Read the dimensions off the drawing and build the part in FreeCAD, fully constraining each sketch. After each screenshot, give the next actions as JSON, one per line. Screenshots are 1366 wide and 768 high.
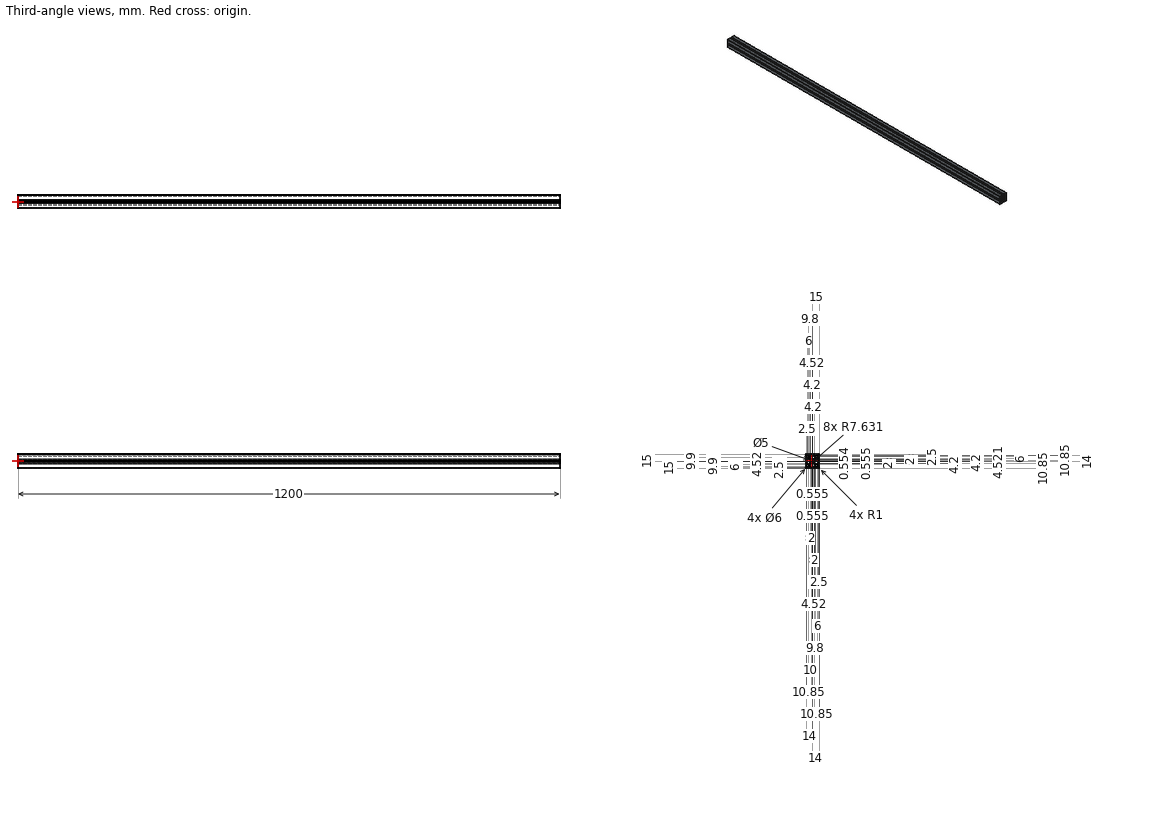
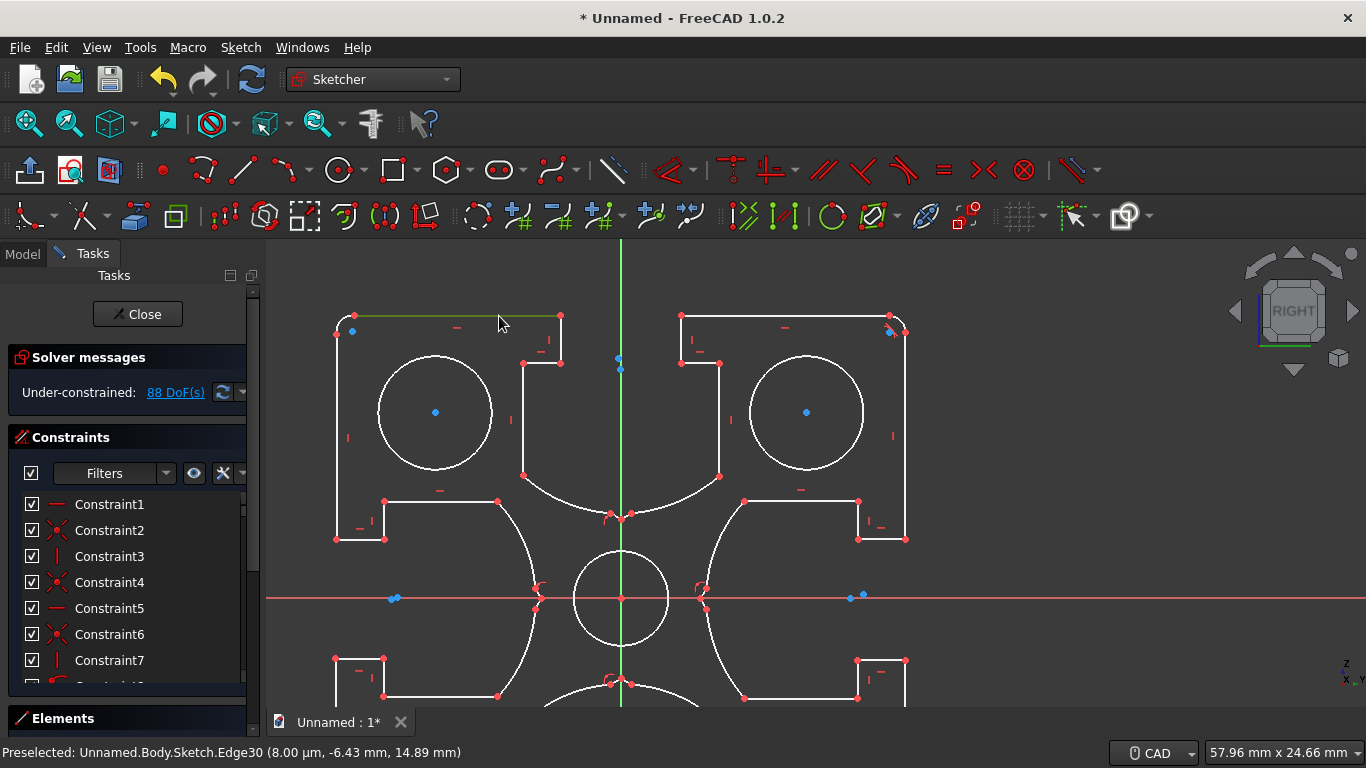
{"action": "left_click", "coordinate": [341, 320]}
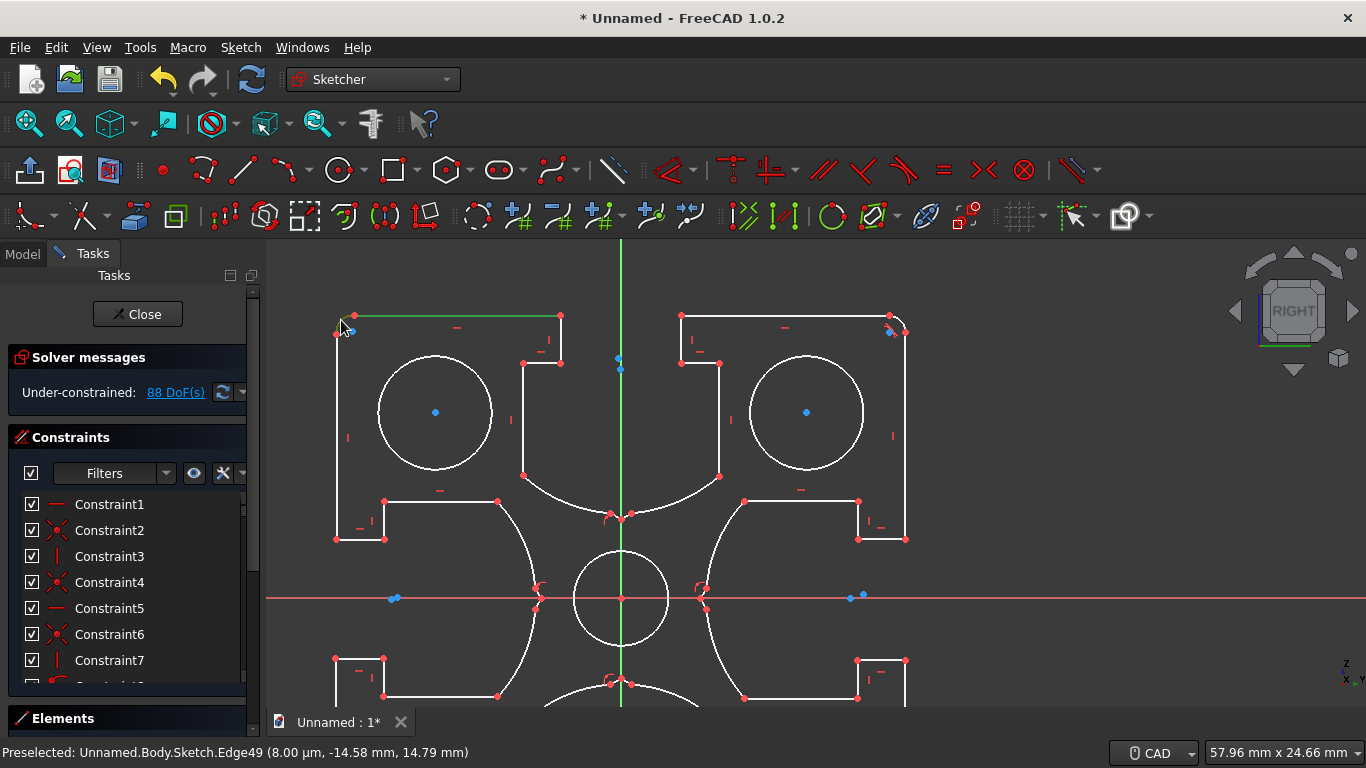
{"action": "left_click", "coordinate": [904, 170]}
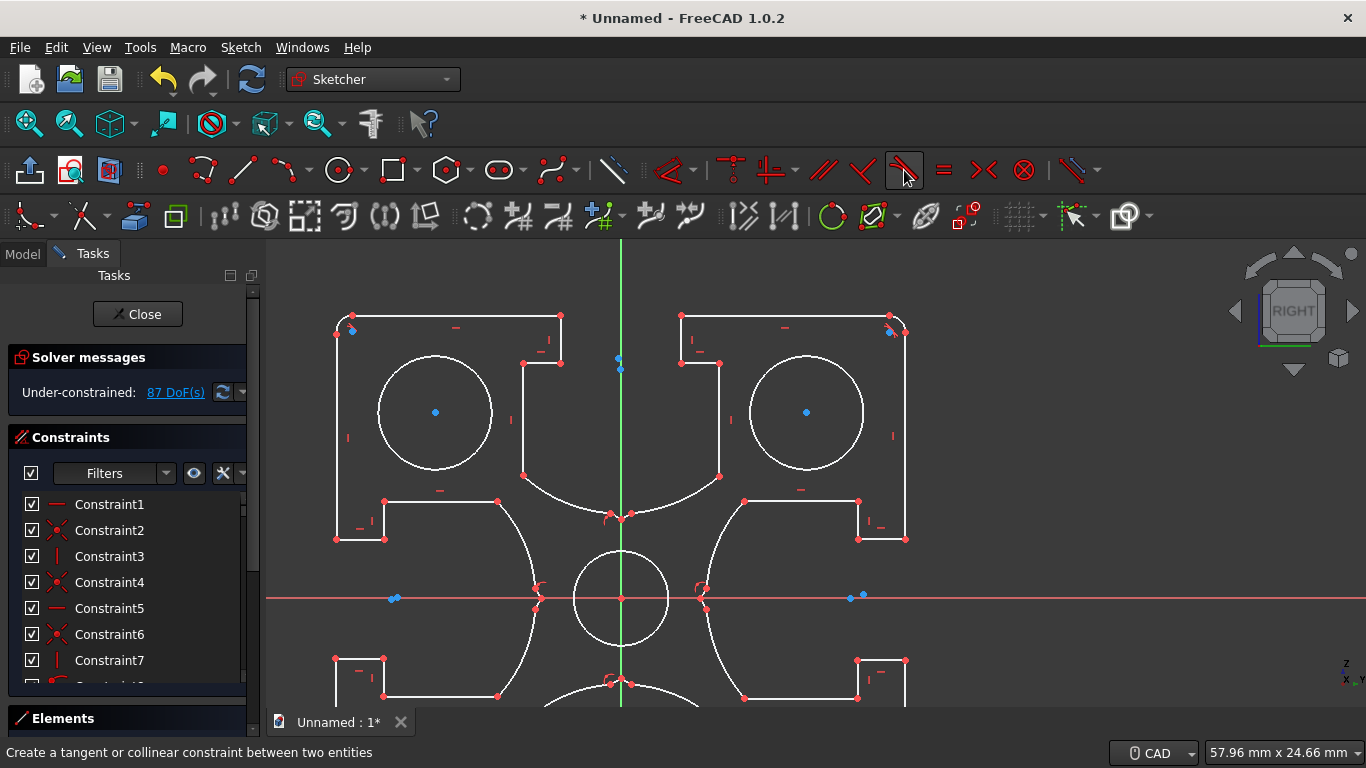
{"action": "left_click", "coordinate": [337, 396]}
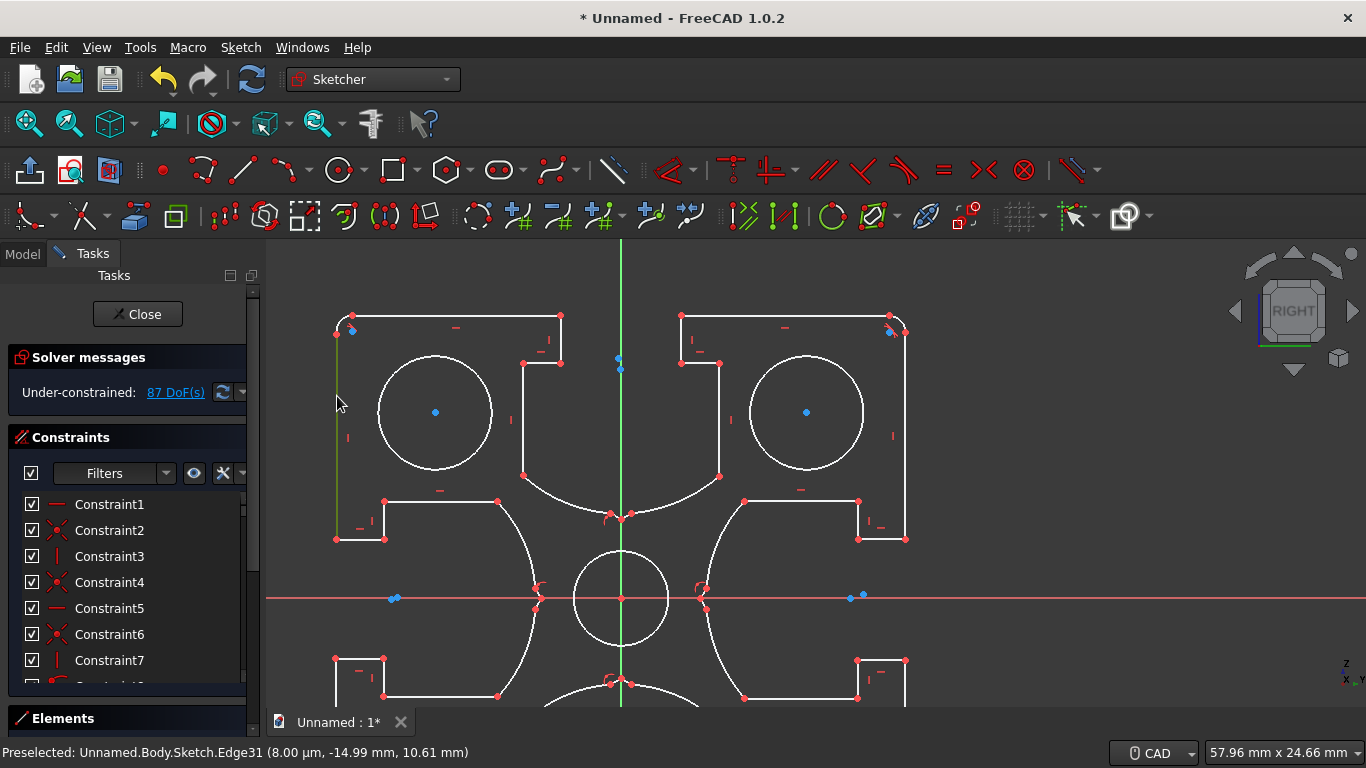
{"action": "left_click", "coordinate": [340, 321]}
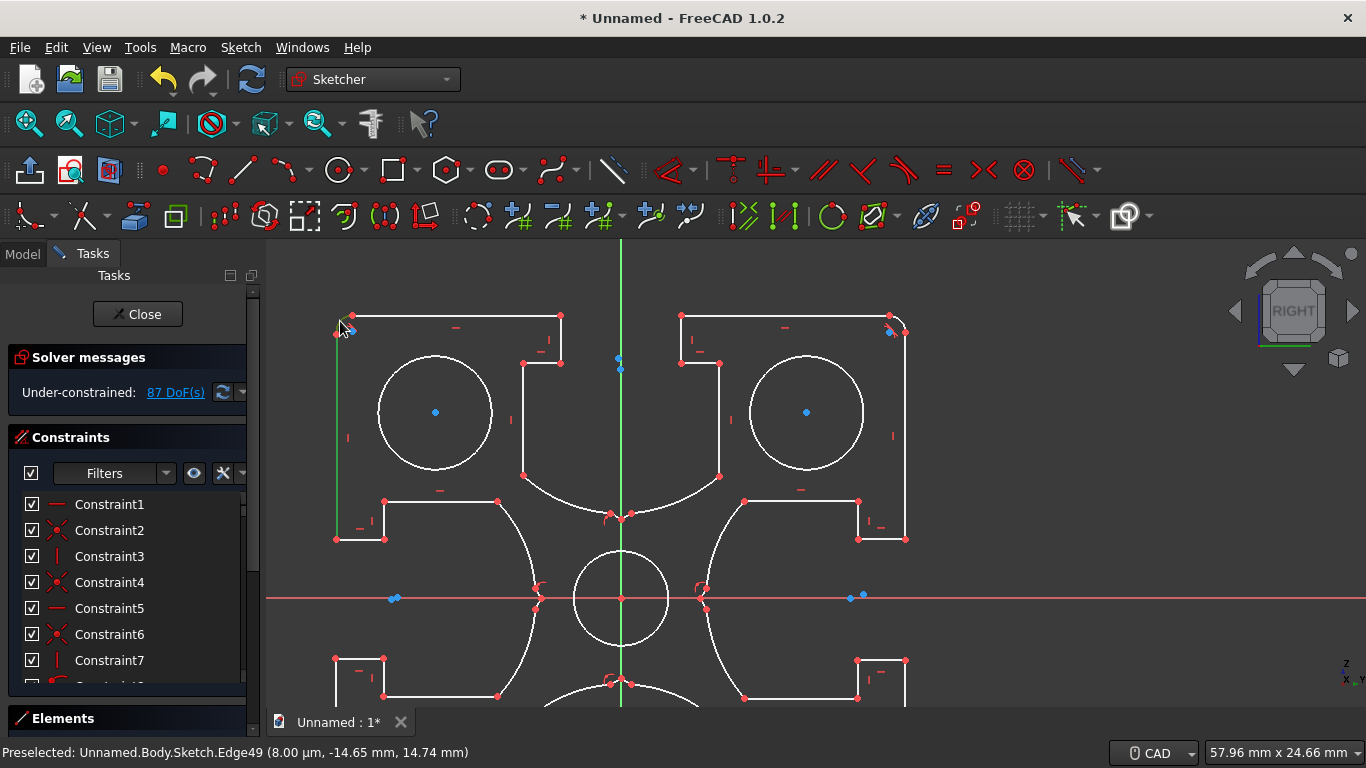
{"action": "left_click", "coordinate": [904, 170]}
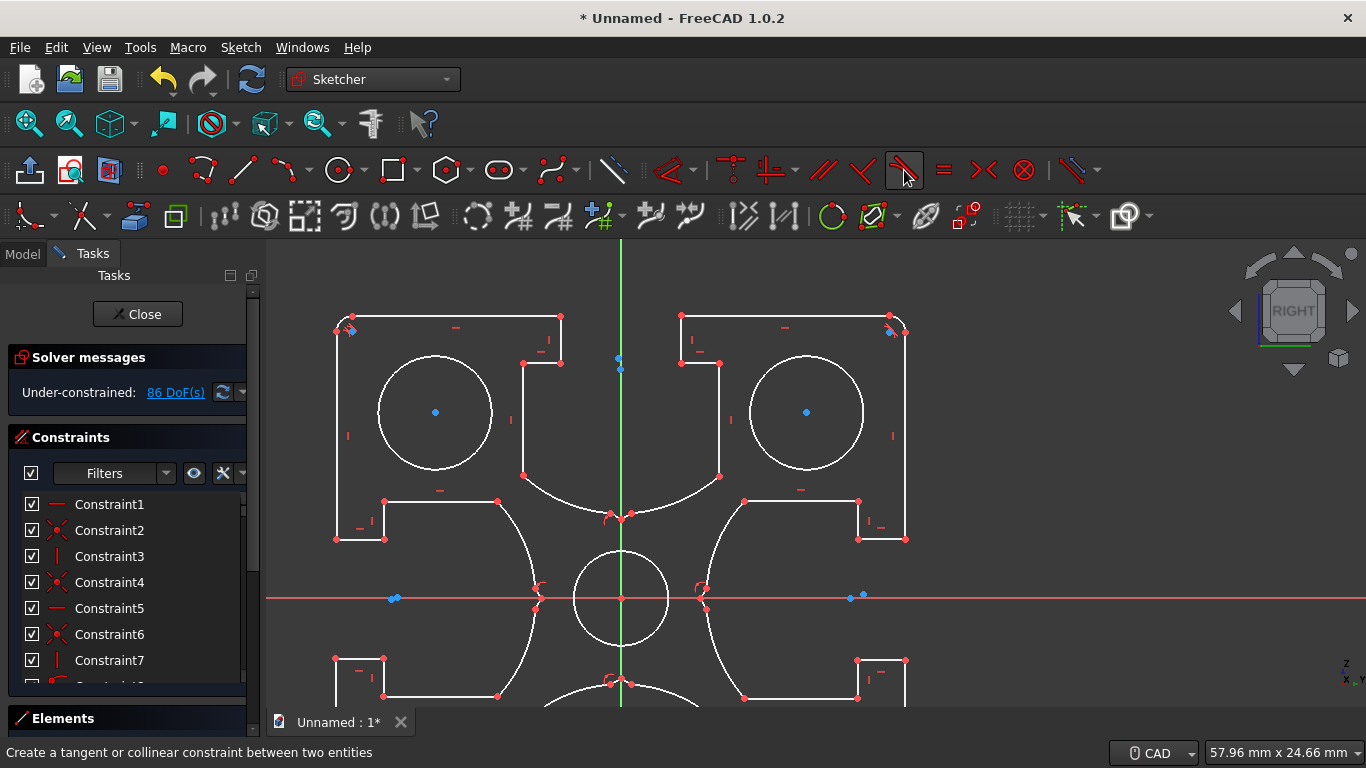
{"action": "scroll", "coordinate": [901, 320], "scroll_direction": "down", "scroll_amount": 3}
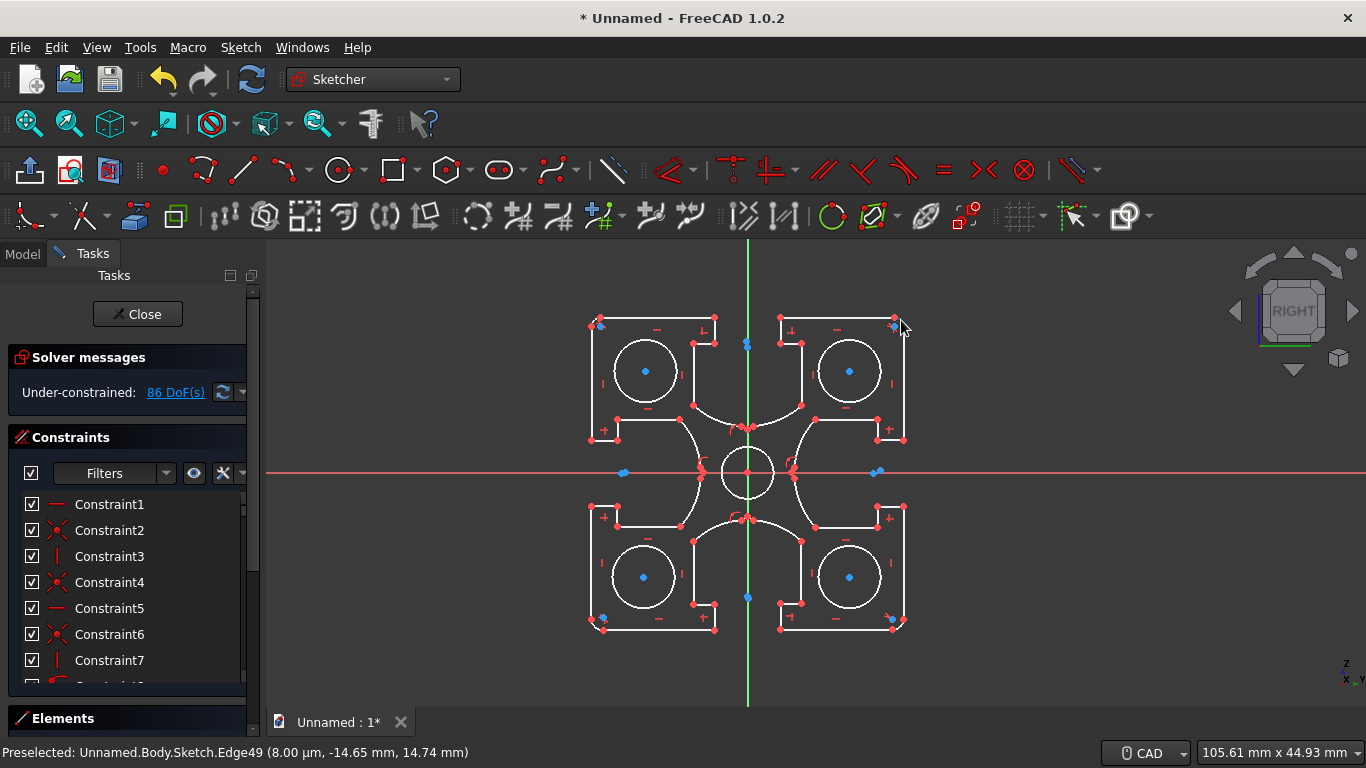
{"action": "left_click", "coordinate": [591, 540]}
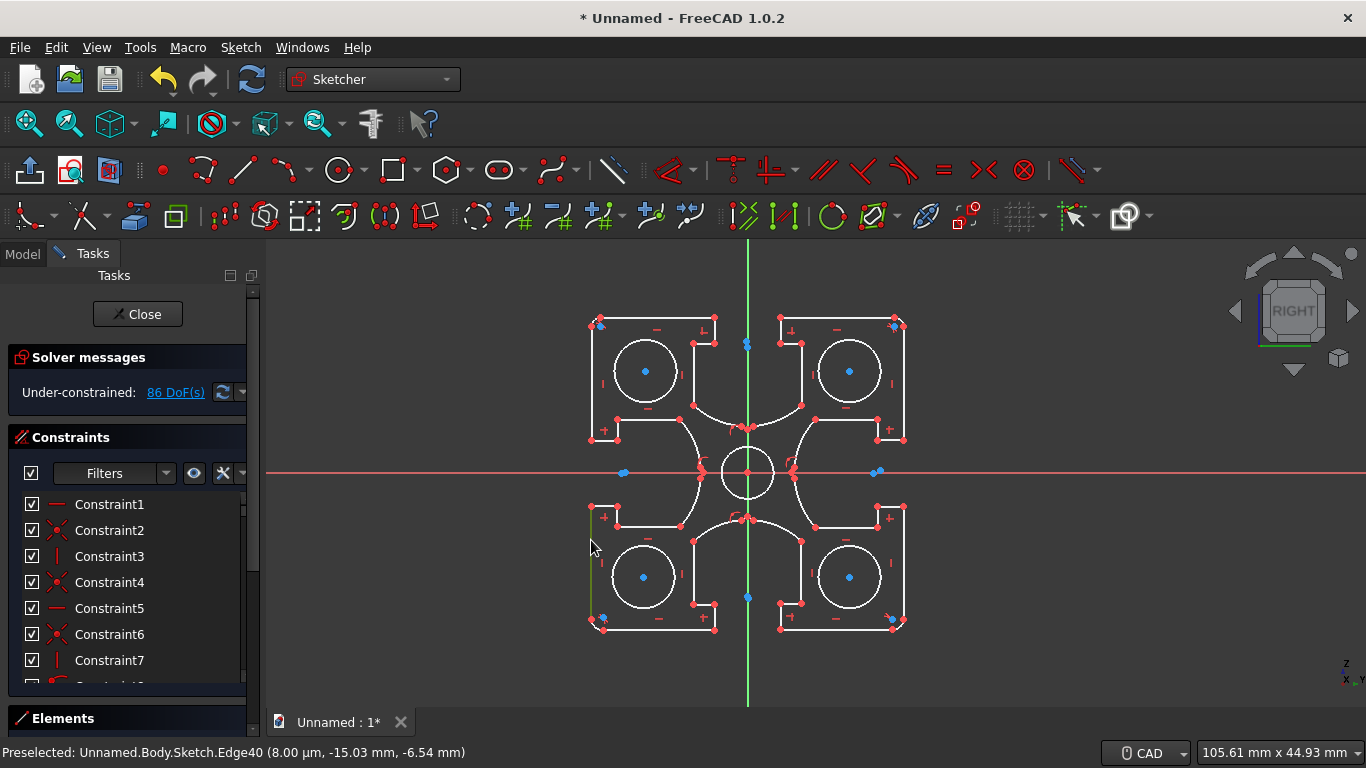
{"action": "scroll", "coordinate": [595, 627], "scroll_direction": "up", "scroll_amount": 3}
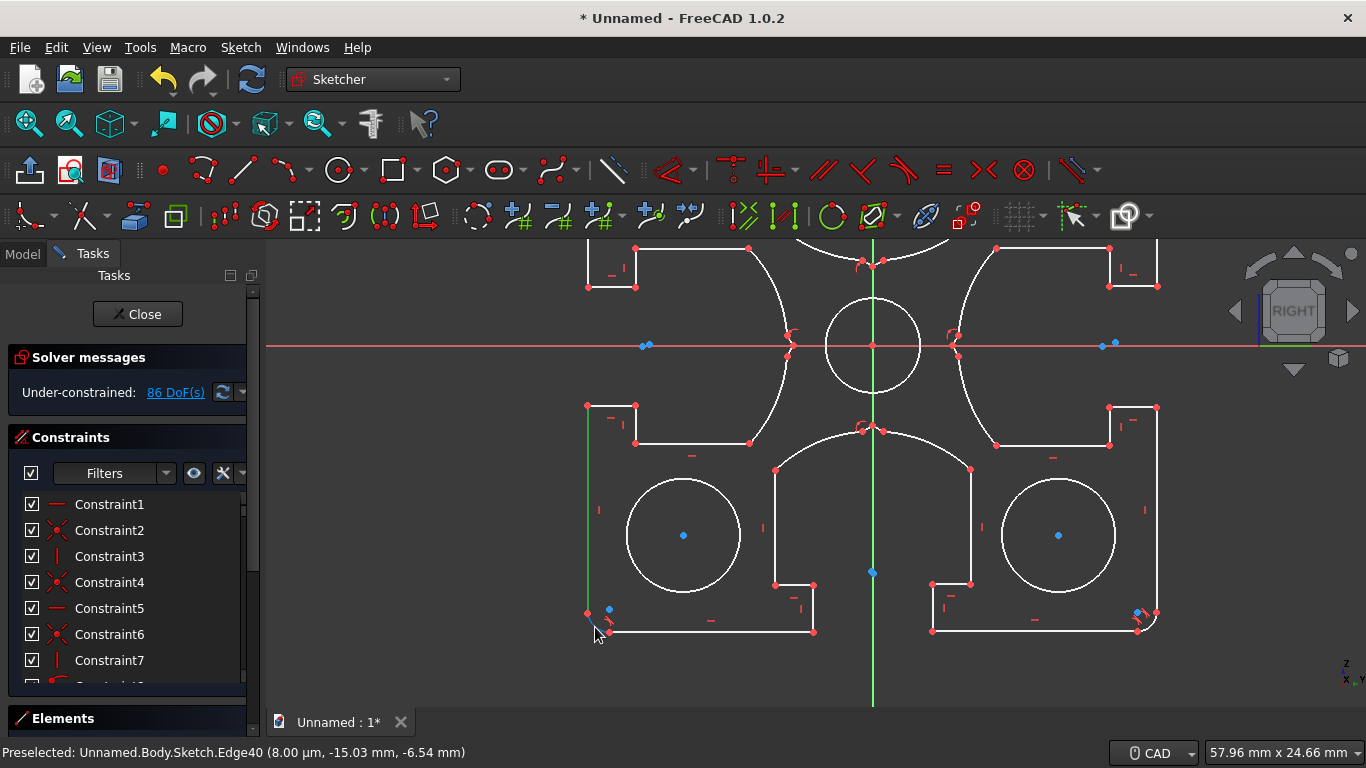
{"action": "left_click", "coordinate": [595, 627]}